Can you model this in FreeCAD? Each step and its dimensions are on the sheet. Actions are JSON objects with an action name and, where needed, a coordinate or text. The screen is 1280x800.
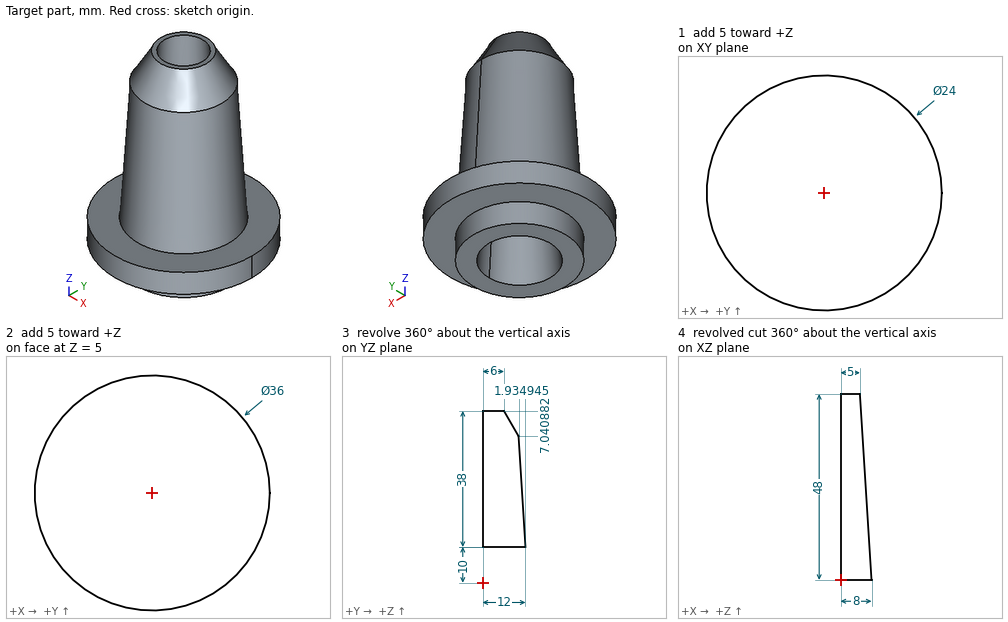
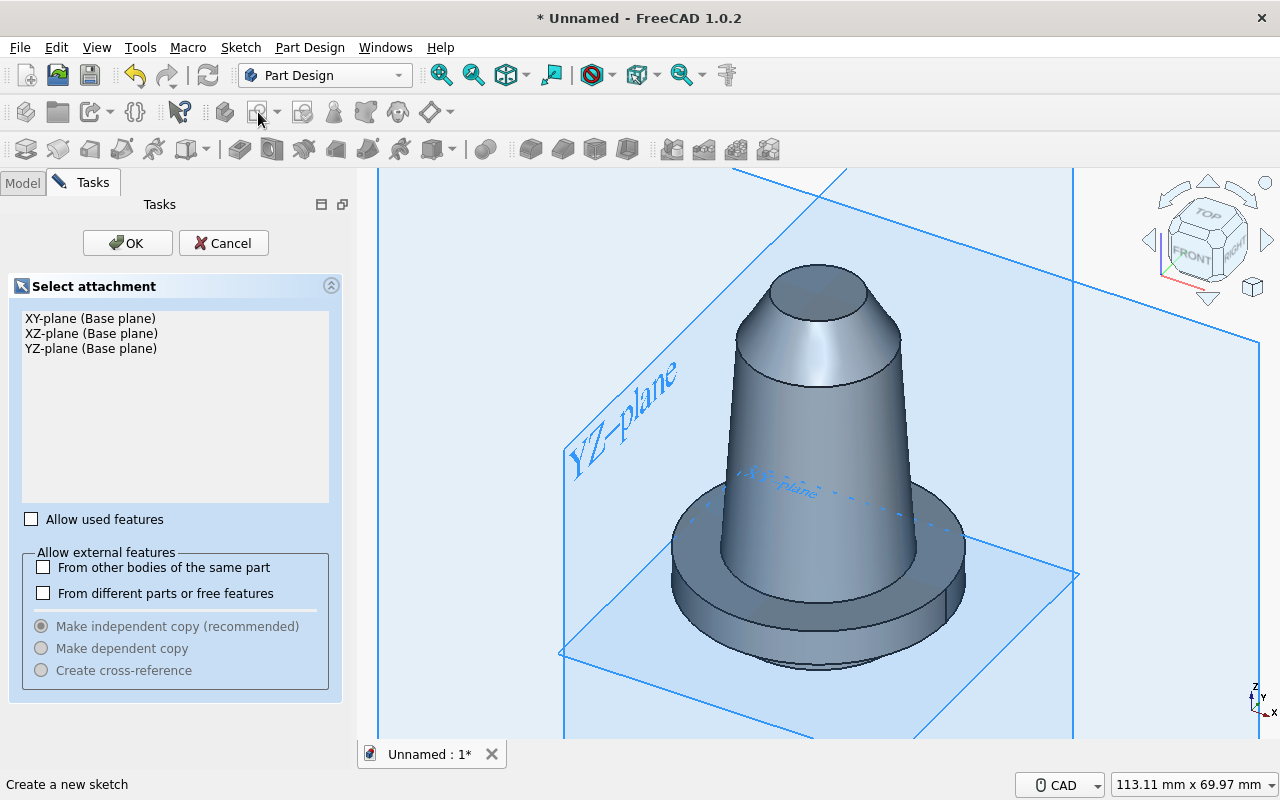
{"action": "left_click", "coordinate": [82, 334]}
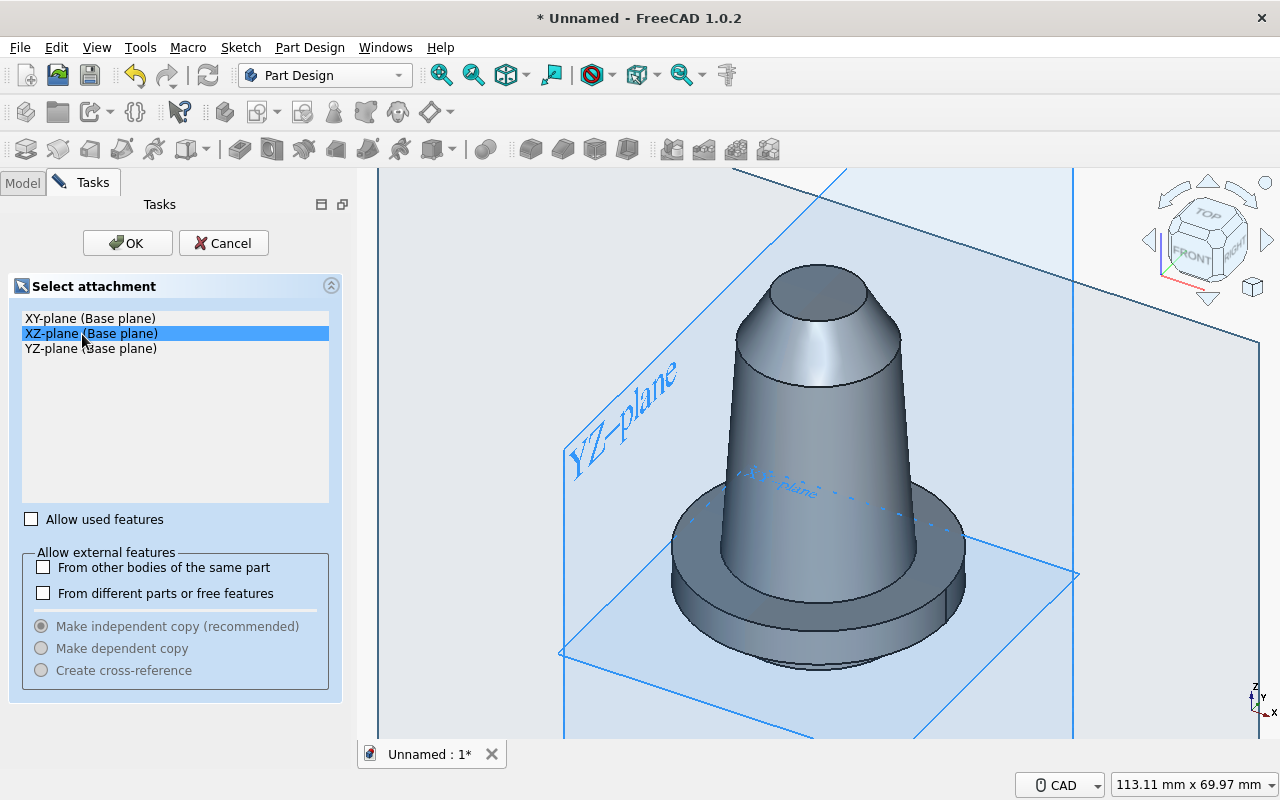
{"action": "left_click", "coordinate": [128, 243]}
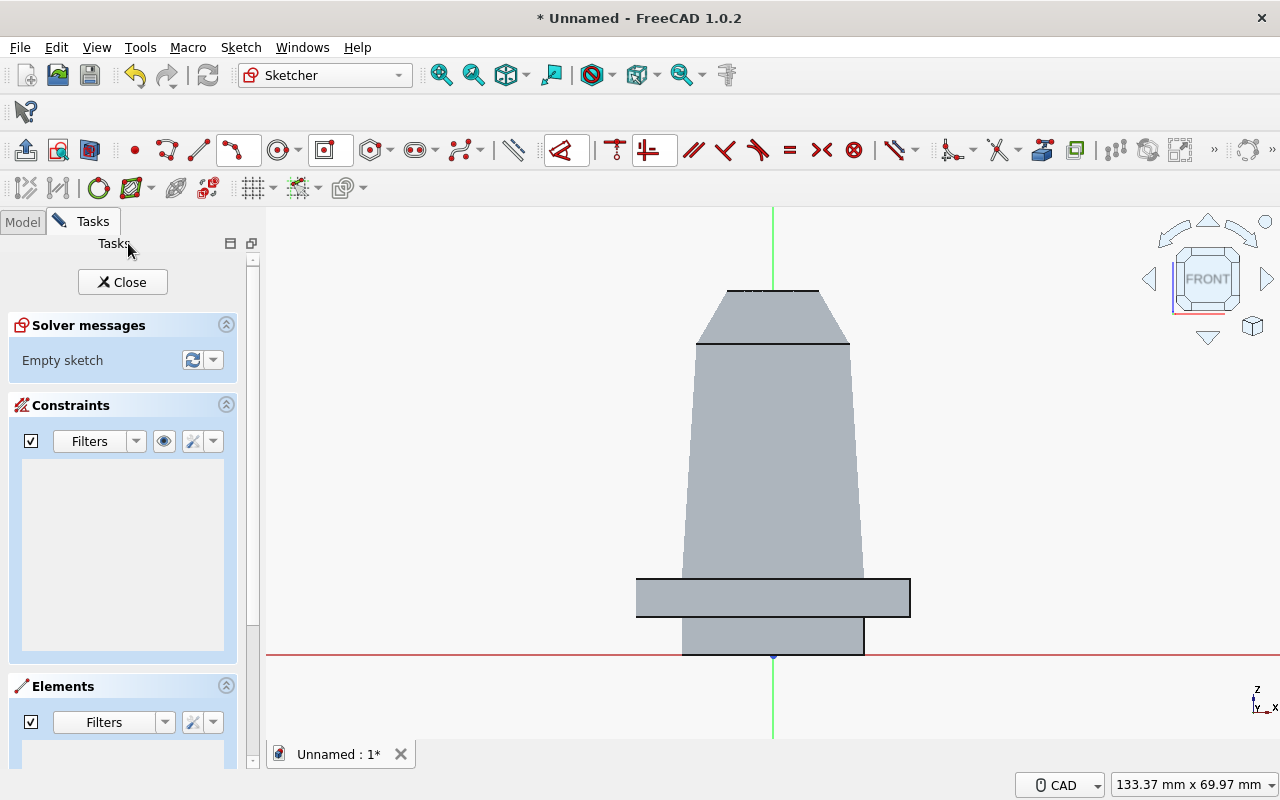
{"action": "left_click", "coordinate": [90, 150]}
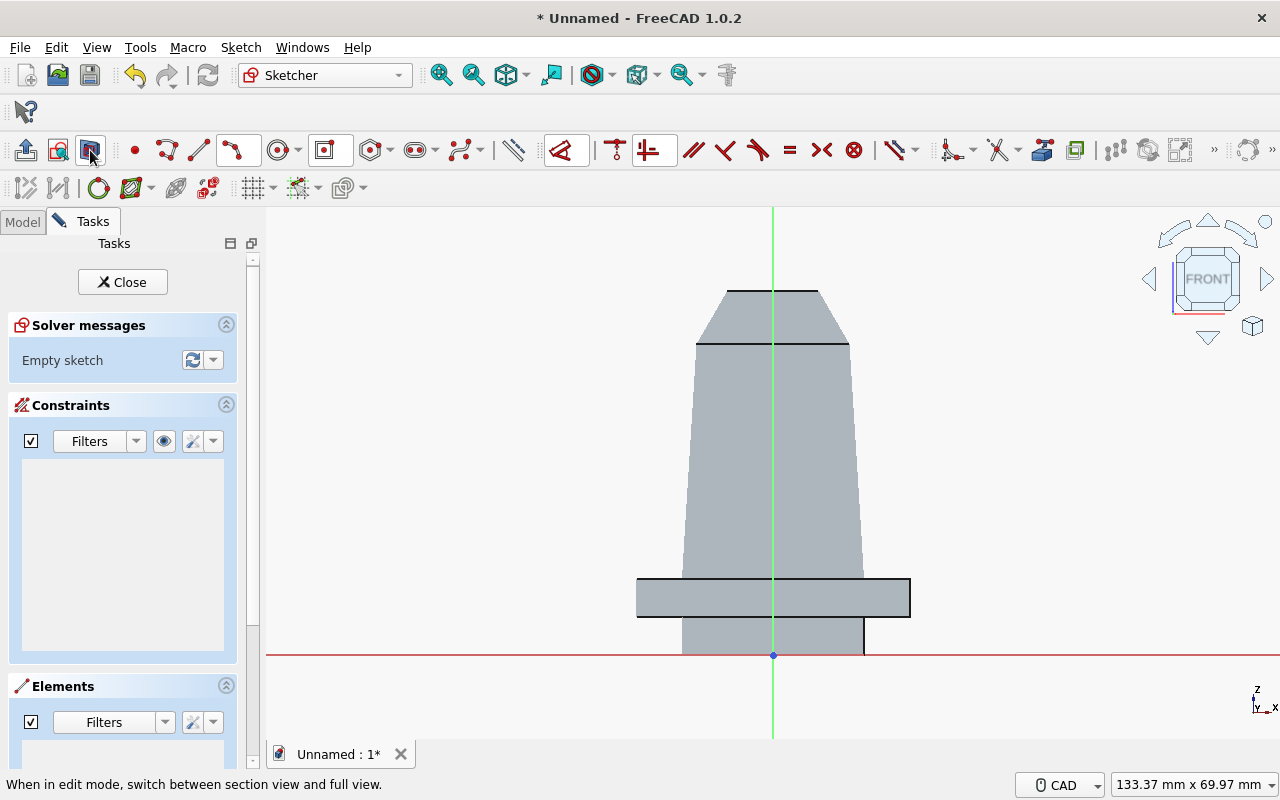
{"action": "left_click", "coordinate": [168, 150]}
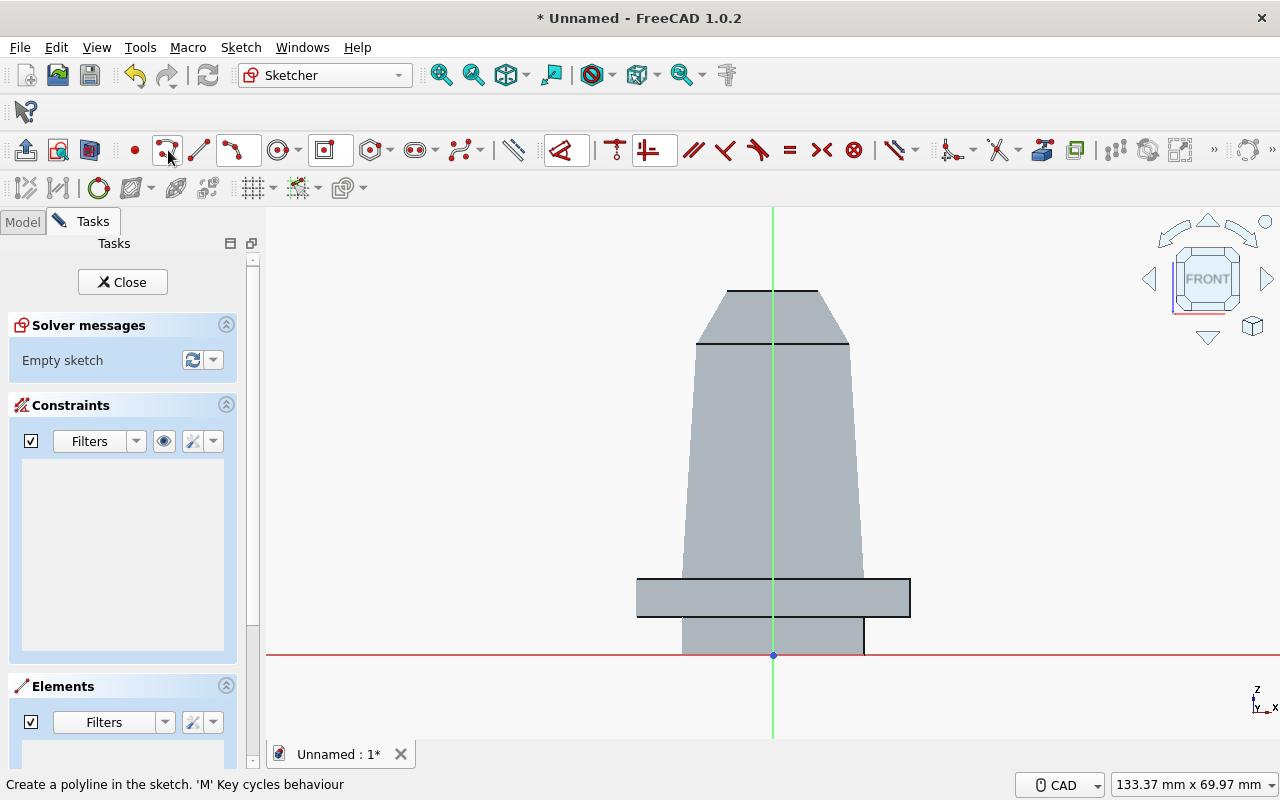
{"action": "left_click", "coordinate": [773, 655]}
{"action": "left_click", "coordinate": [782, 291]}
{"action": "left_click", "coordinate": [811, 291]}
{"action": "left_click", "coordinate": [834, 646]}
{"action": "left_click", "coordinate": [773, 655]}
{"action": "key", "text": "Escape"}
{"action": "key", "text": "Escape"}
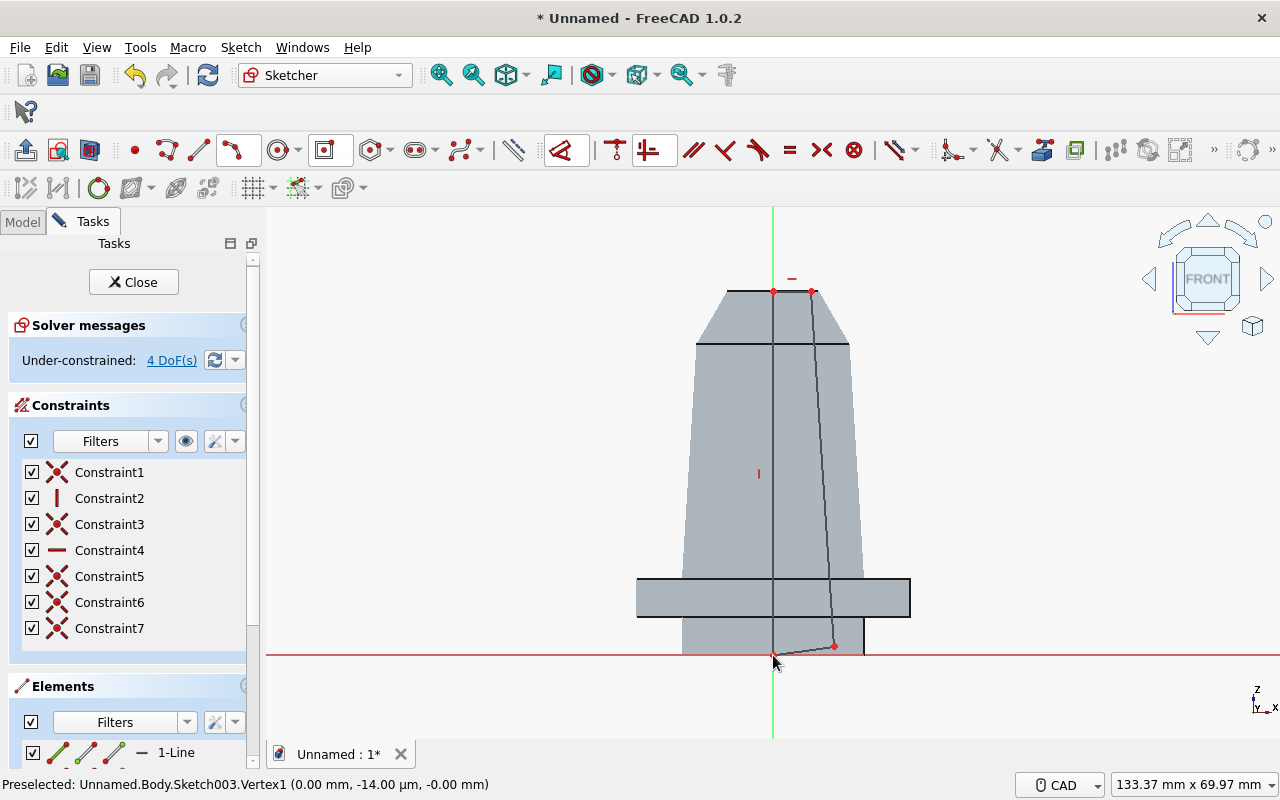
{"action": "left_click", "coordinate": [791, 653]}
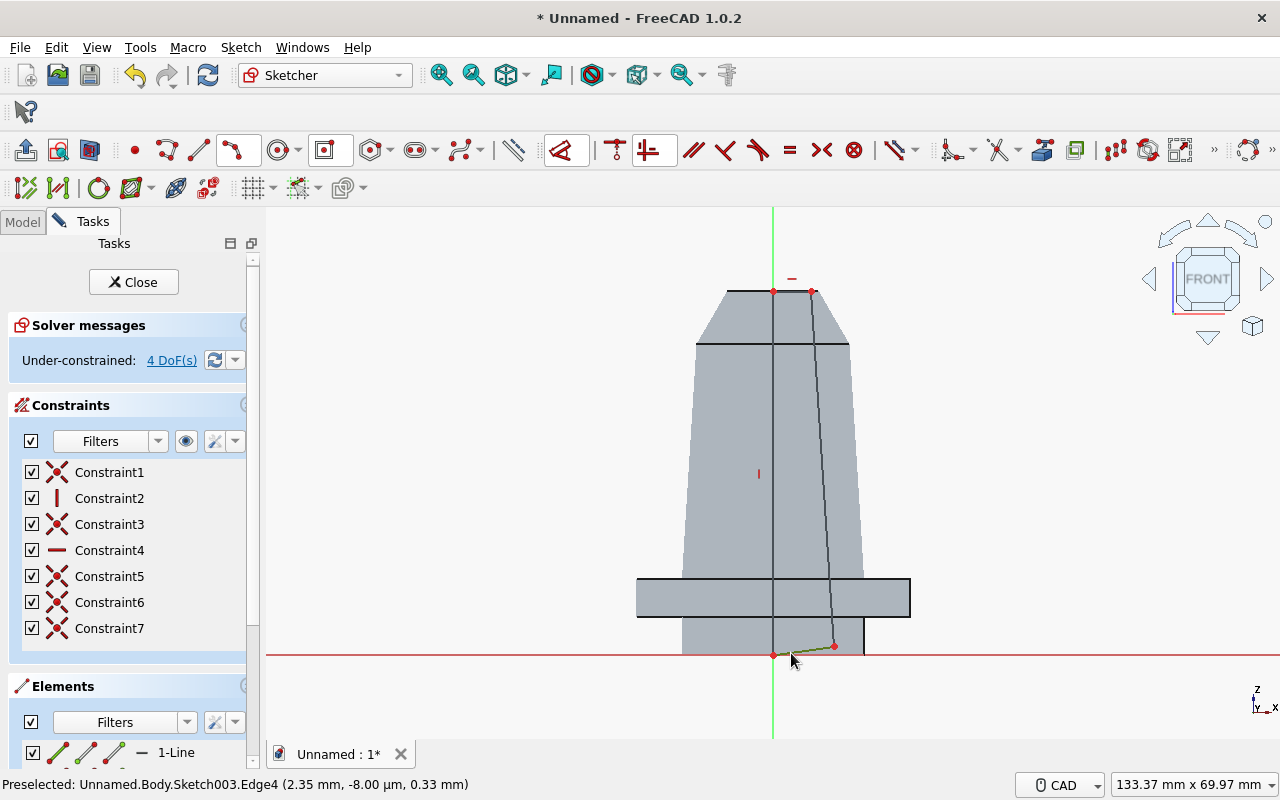
{"action": "left_click", "coordinate": [672, 150]}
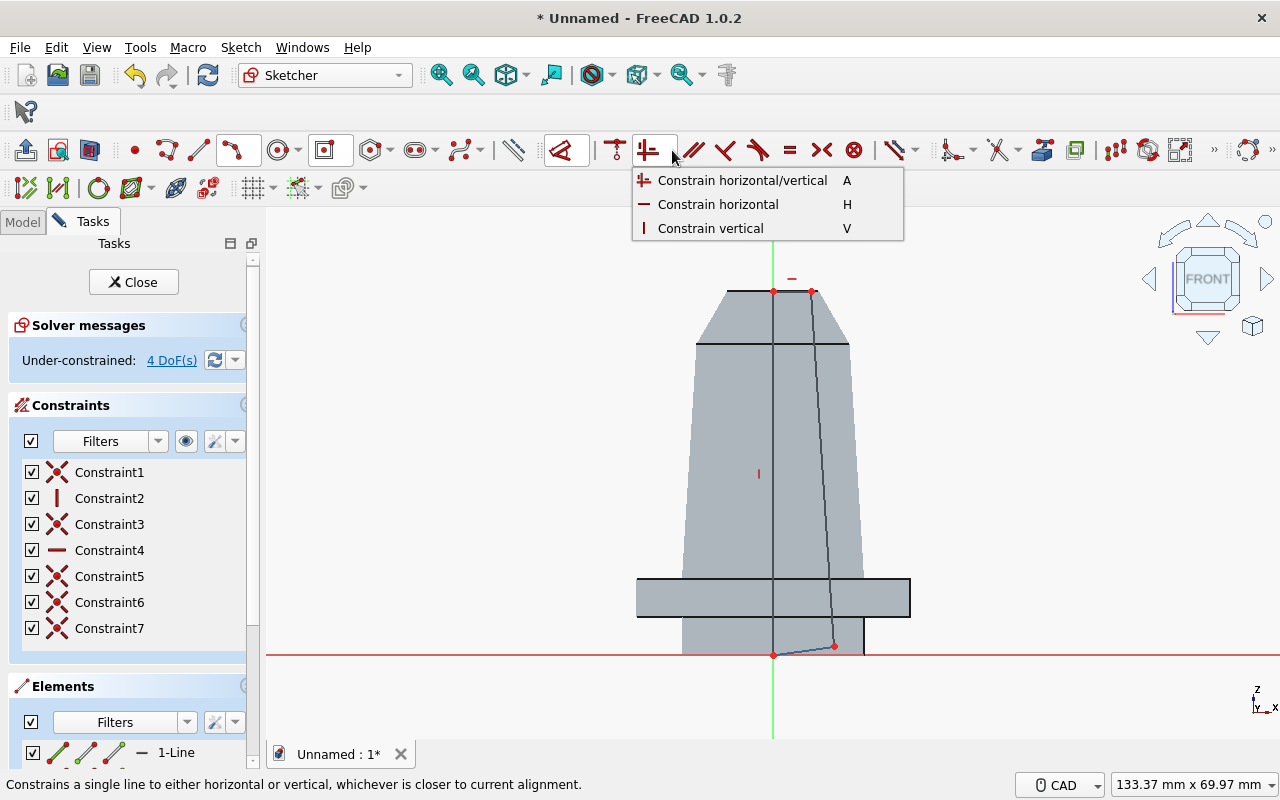
{"action": "left_click", "coordinate": [768, 204]}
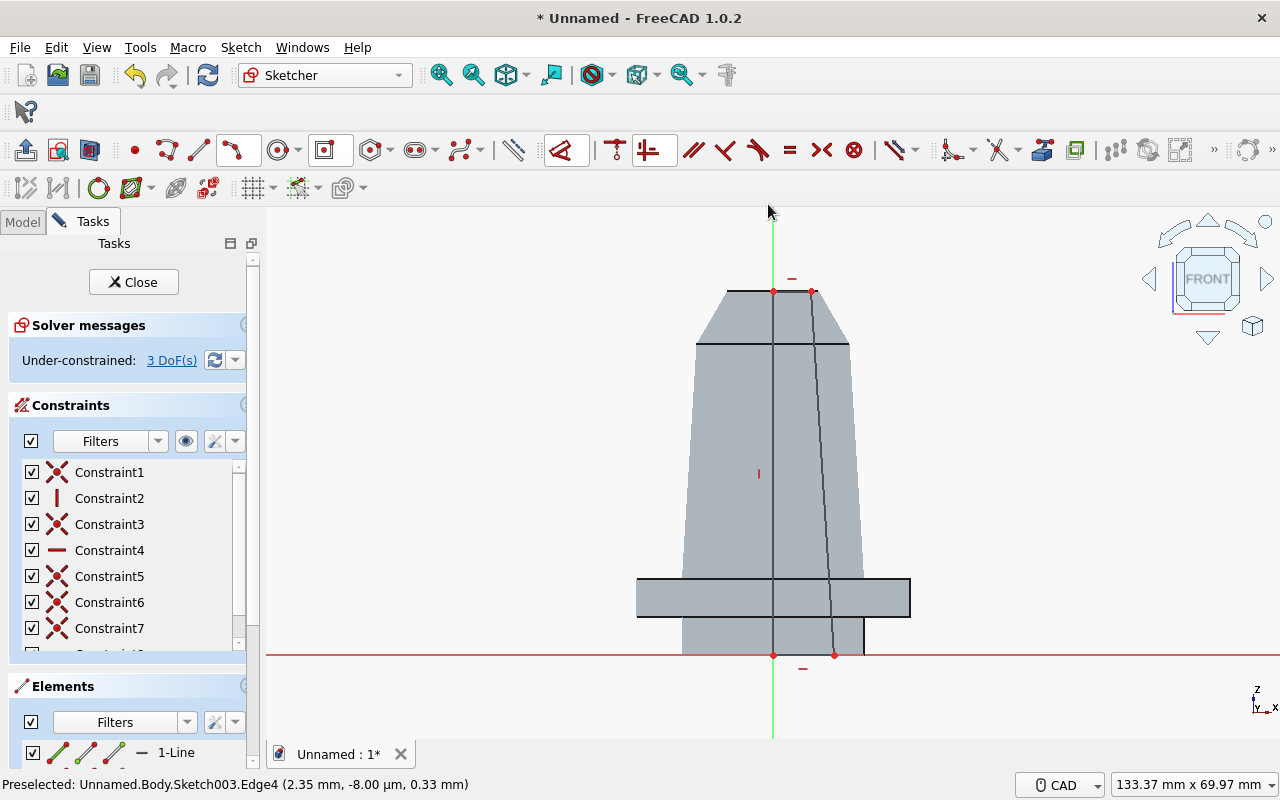
{"action": "left_click", "coordinate": [784, 292]}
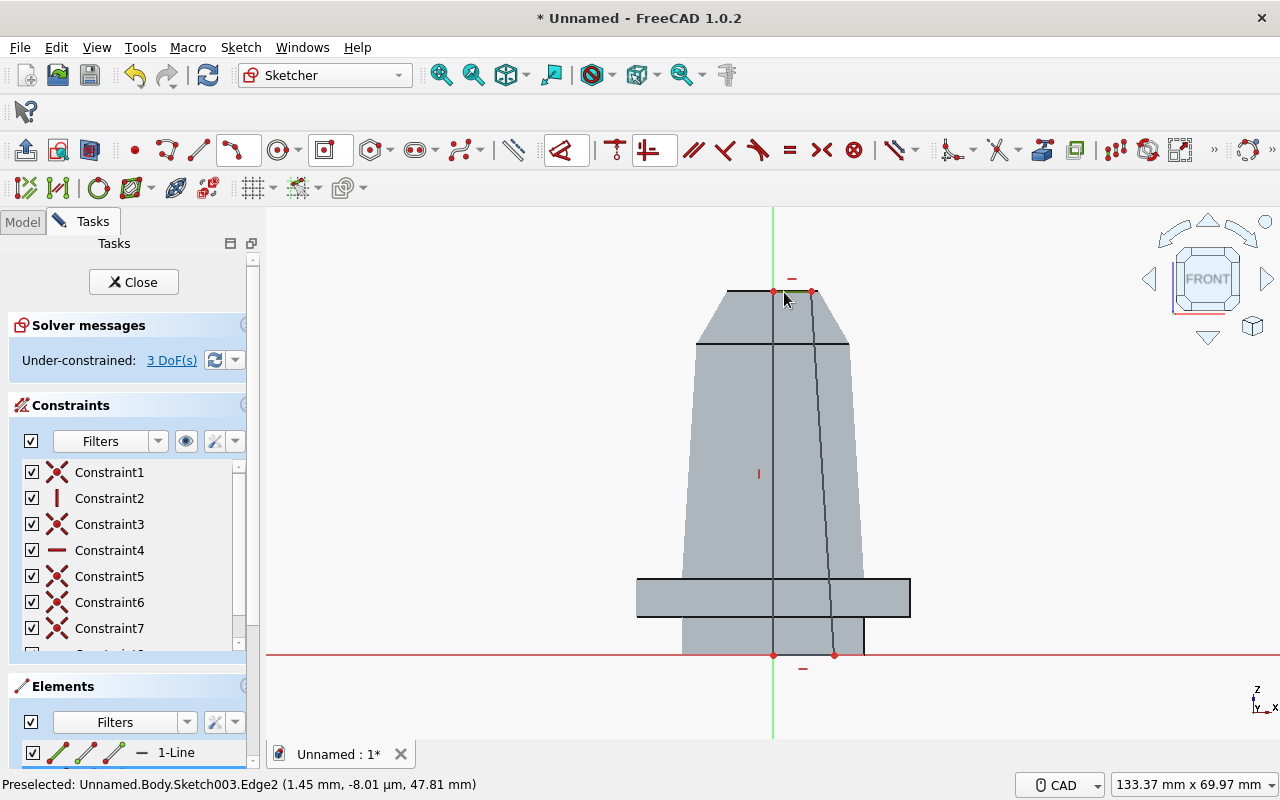
{"action": "left_click", "coordinate": [584, 150]}